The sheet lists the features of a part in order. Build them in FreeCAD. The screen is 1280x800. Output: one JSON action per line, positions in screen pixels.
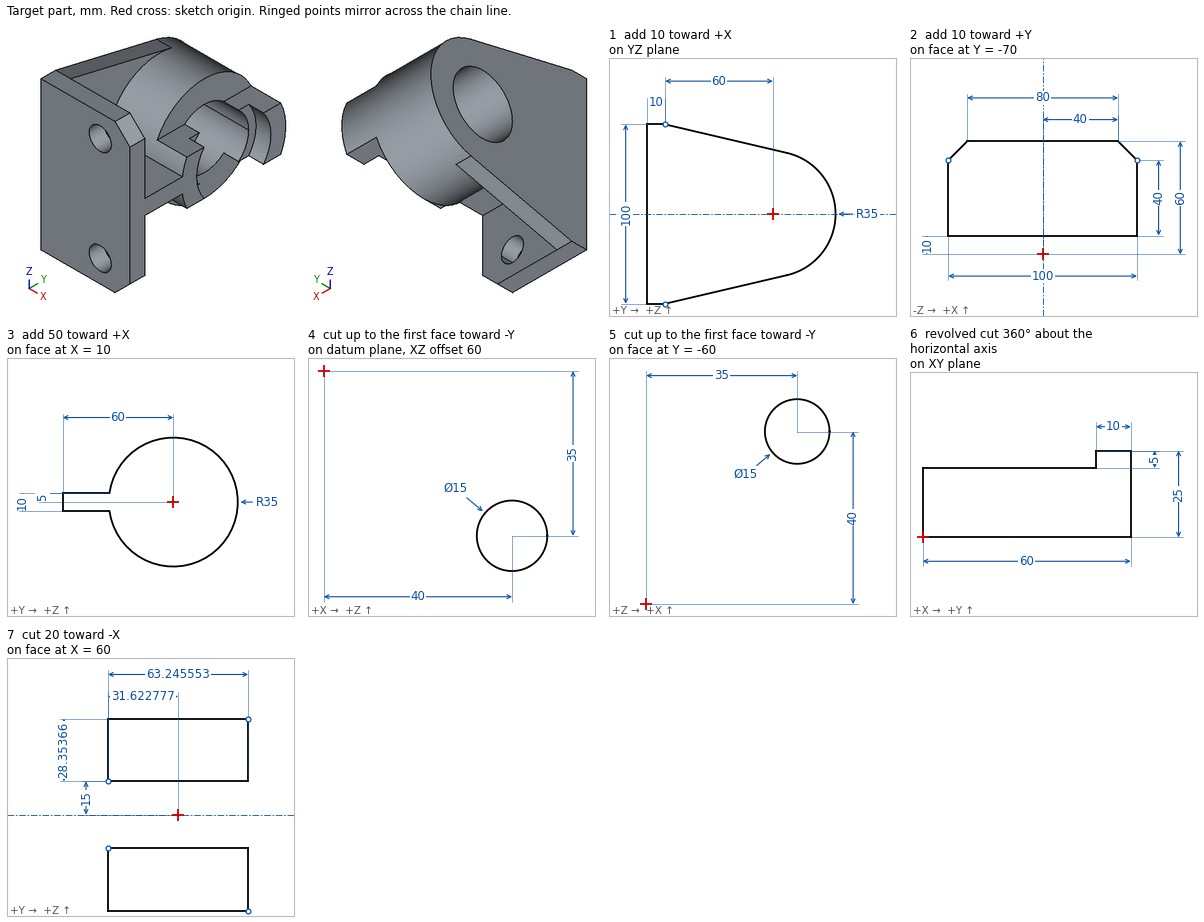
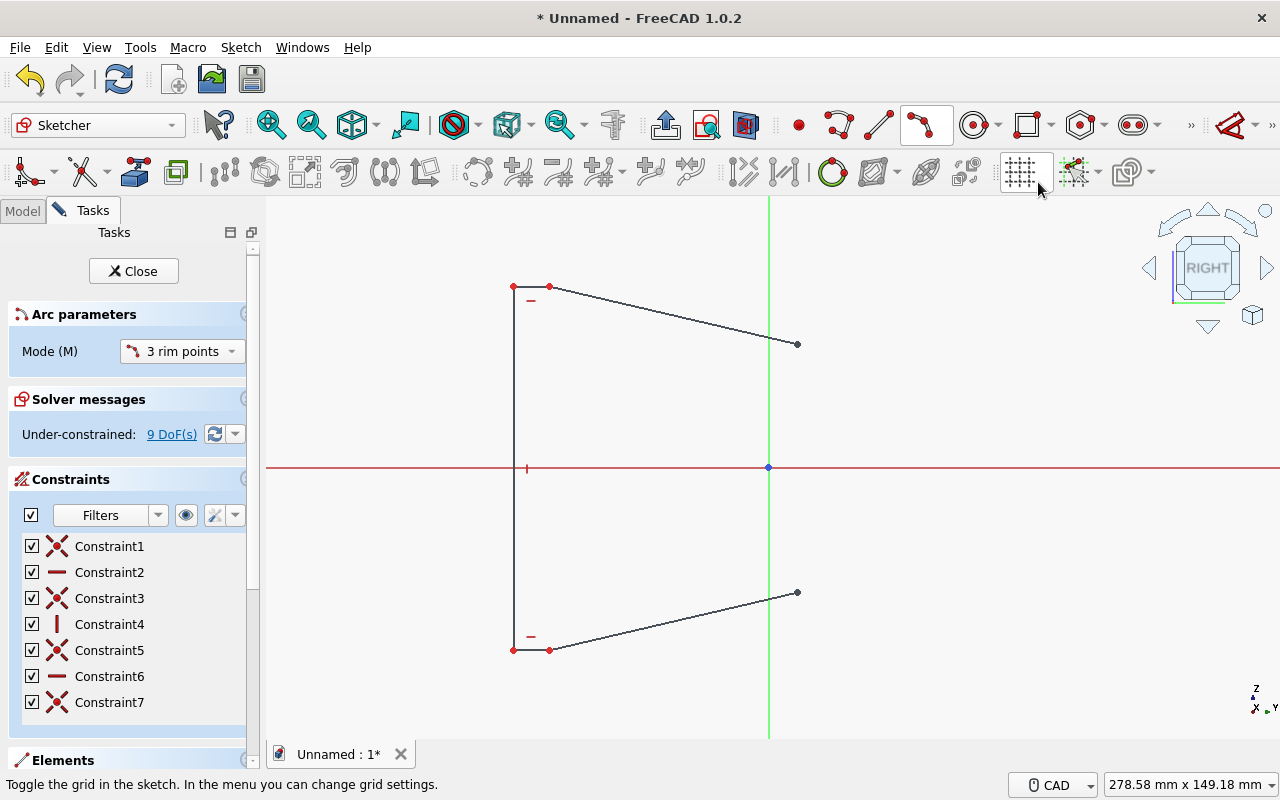
{"action": "left_click", "coordinate": [798, 593]}
{"action": "left_click", "coordinate": [798, 344]}
{"action": "left_click", "coordinate": [891, 501]}
{"action": "key", "text": "Escape"}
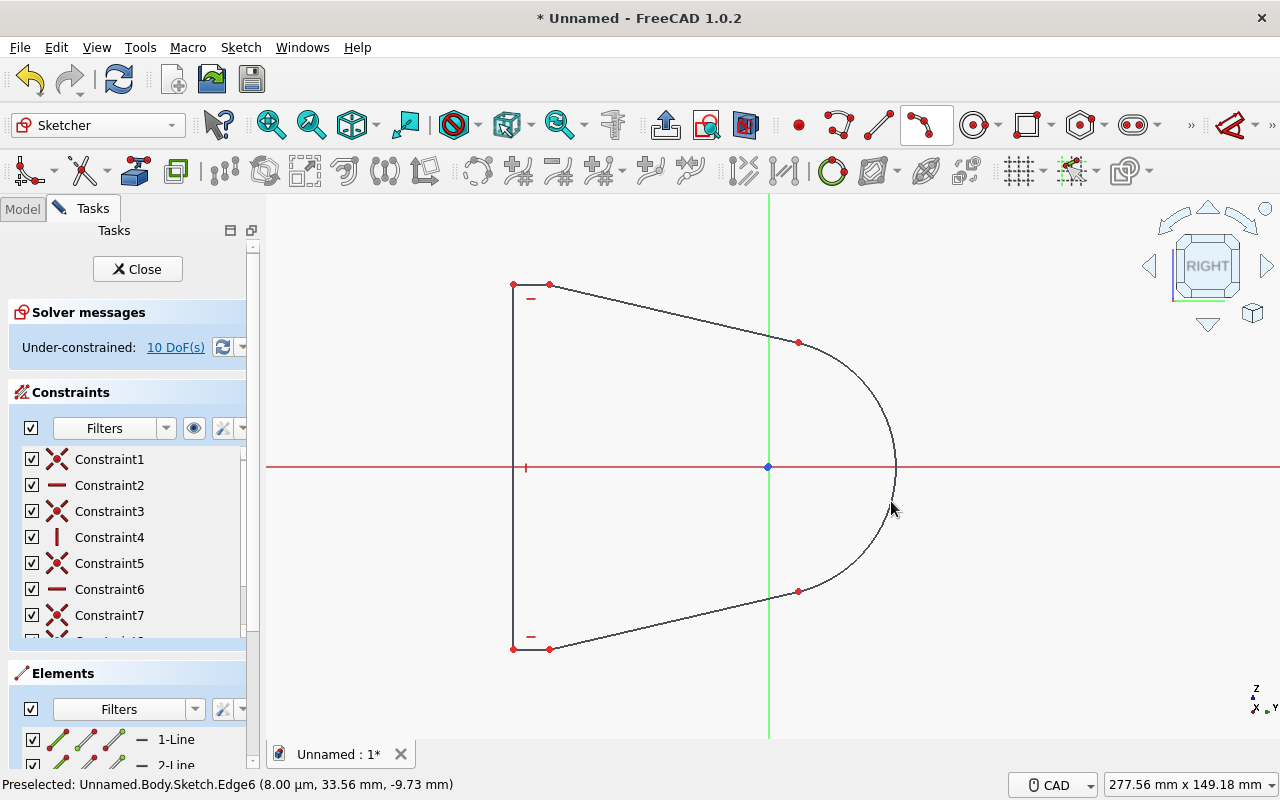
{"action": "left_click", "coordinate": [723, 326]}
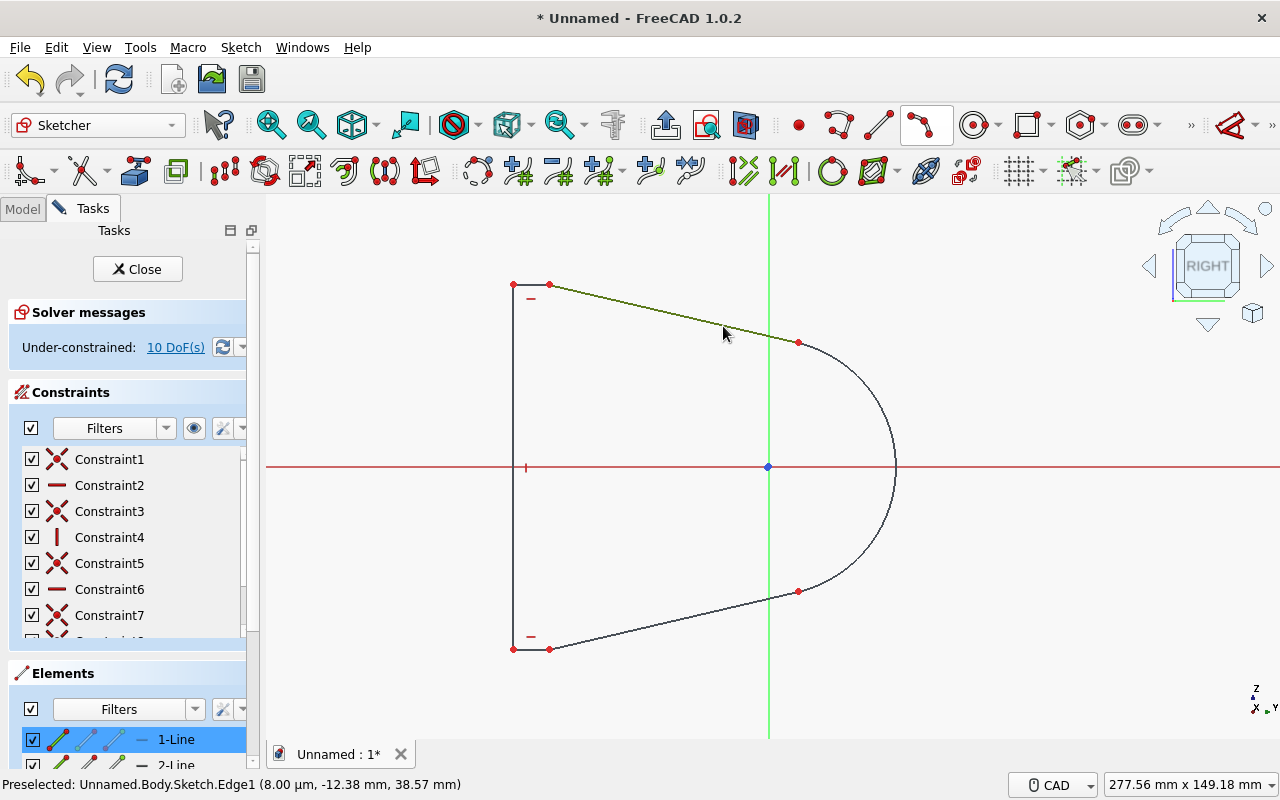
{"action": "left_click", "coordinate": [878, 533]}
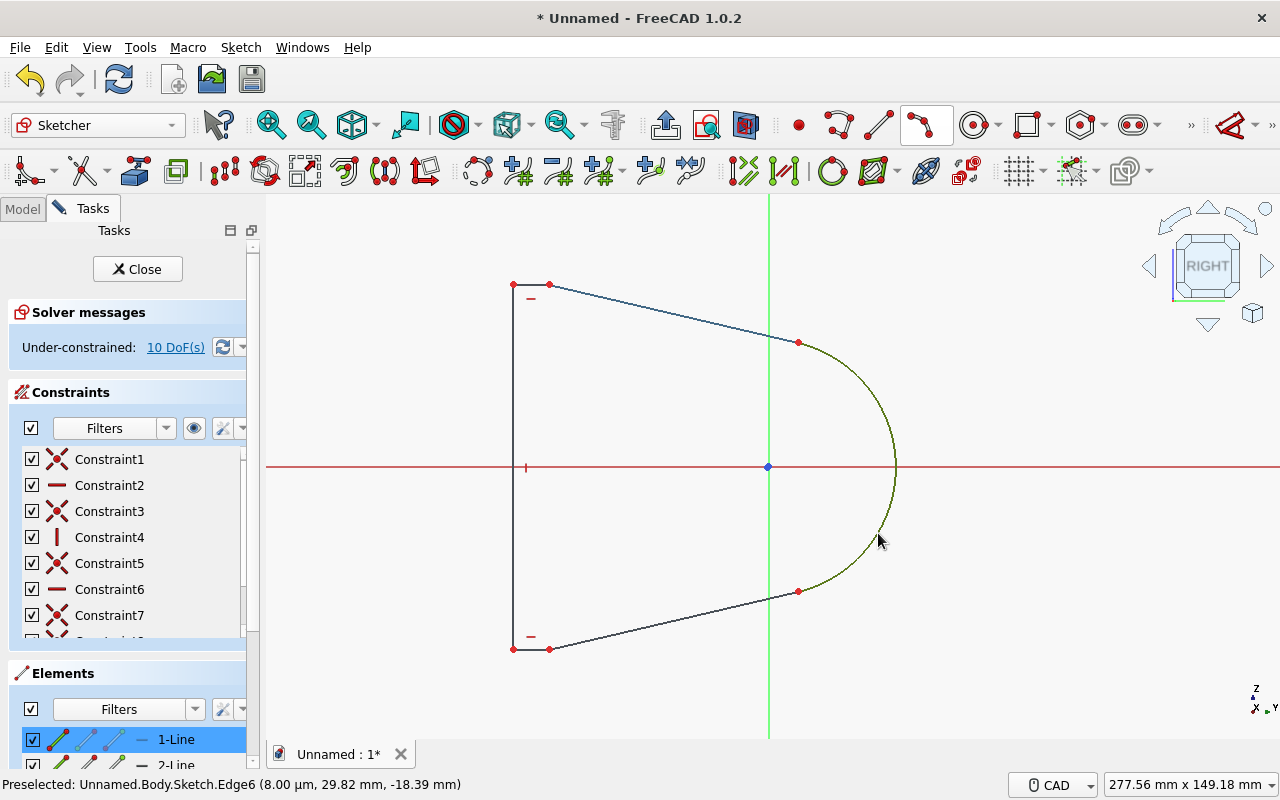
{"action": "key", "text": "t"}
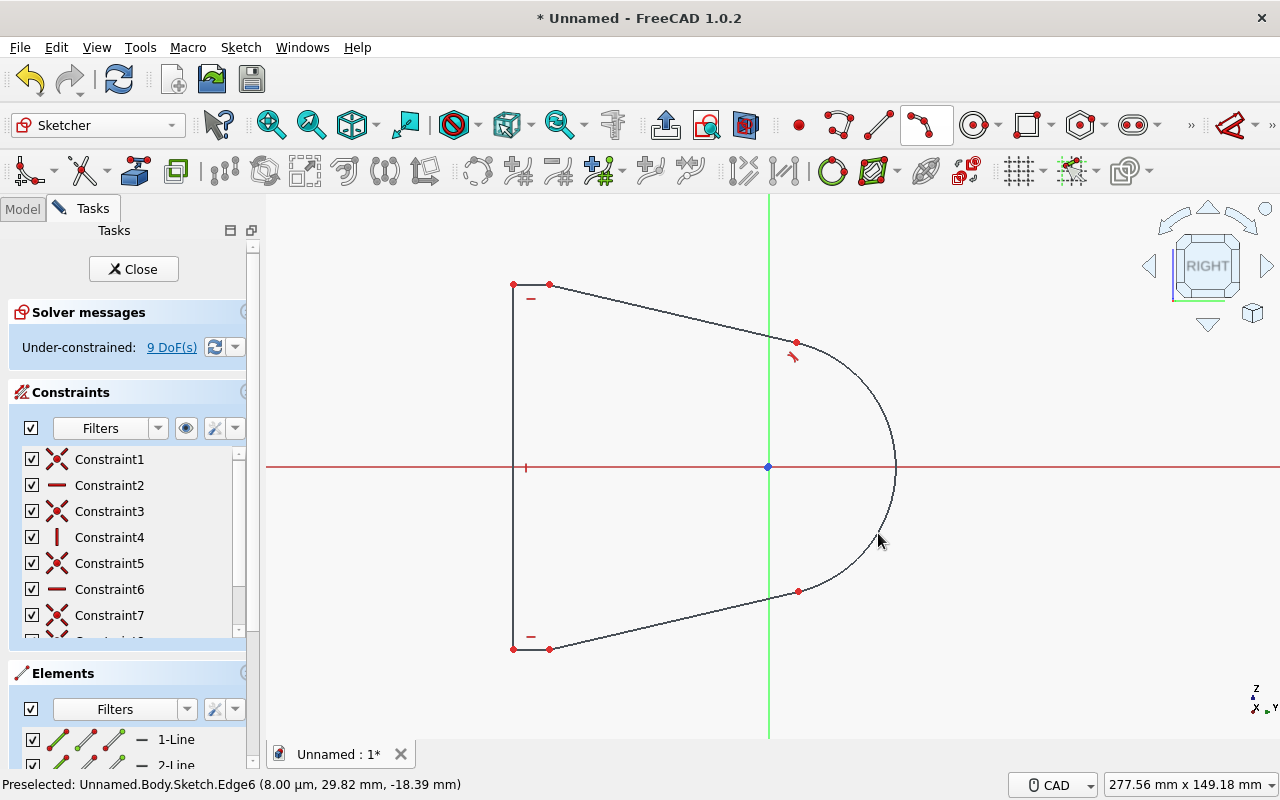
{"action": "left_click", "coordinate": [624, 633]}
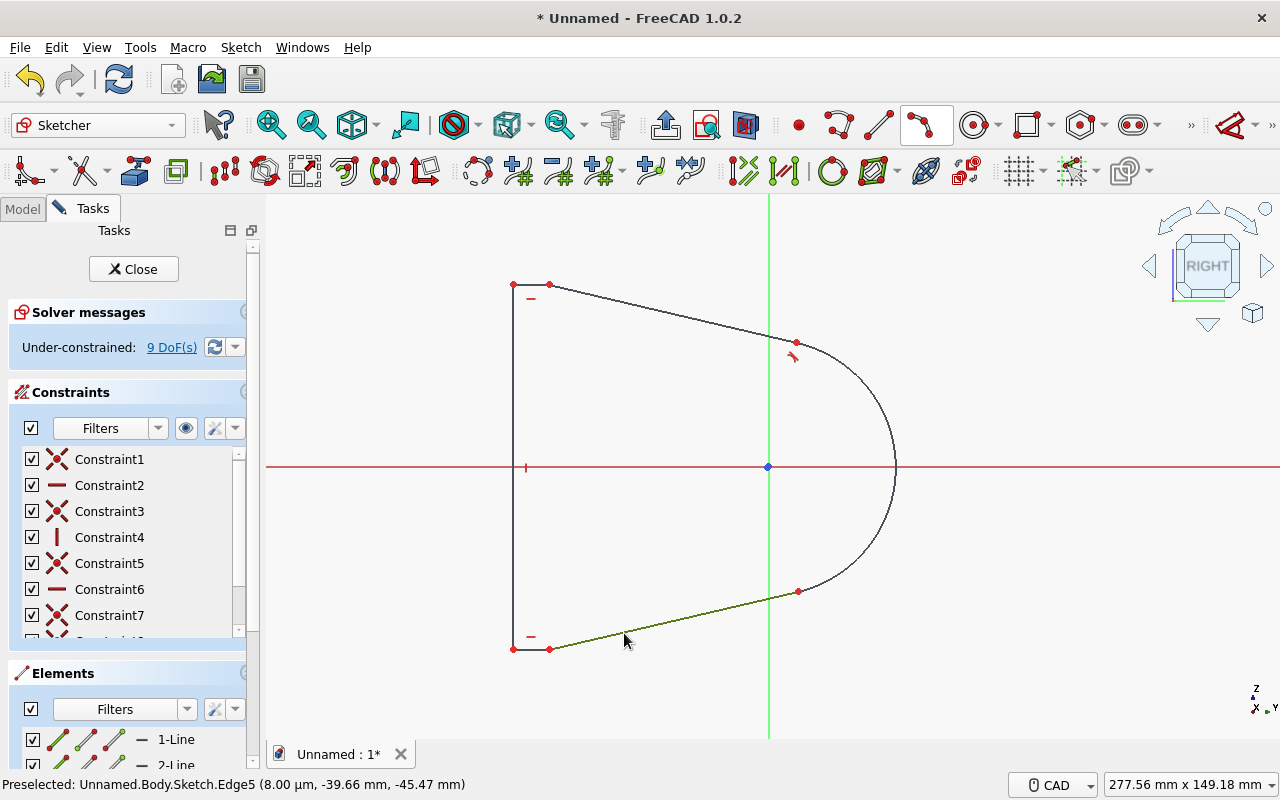
{"action": "left_click", "coordinate": [878, 532]}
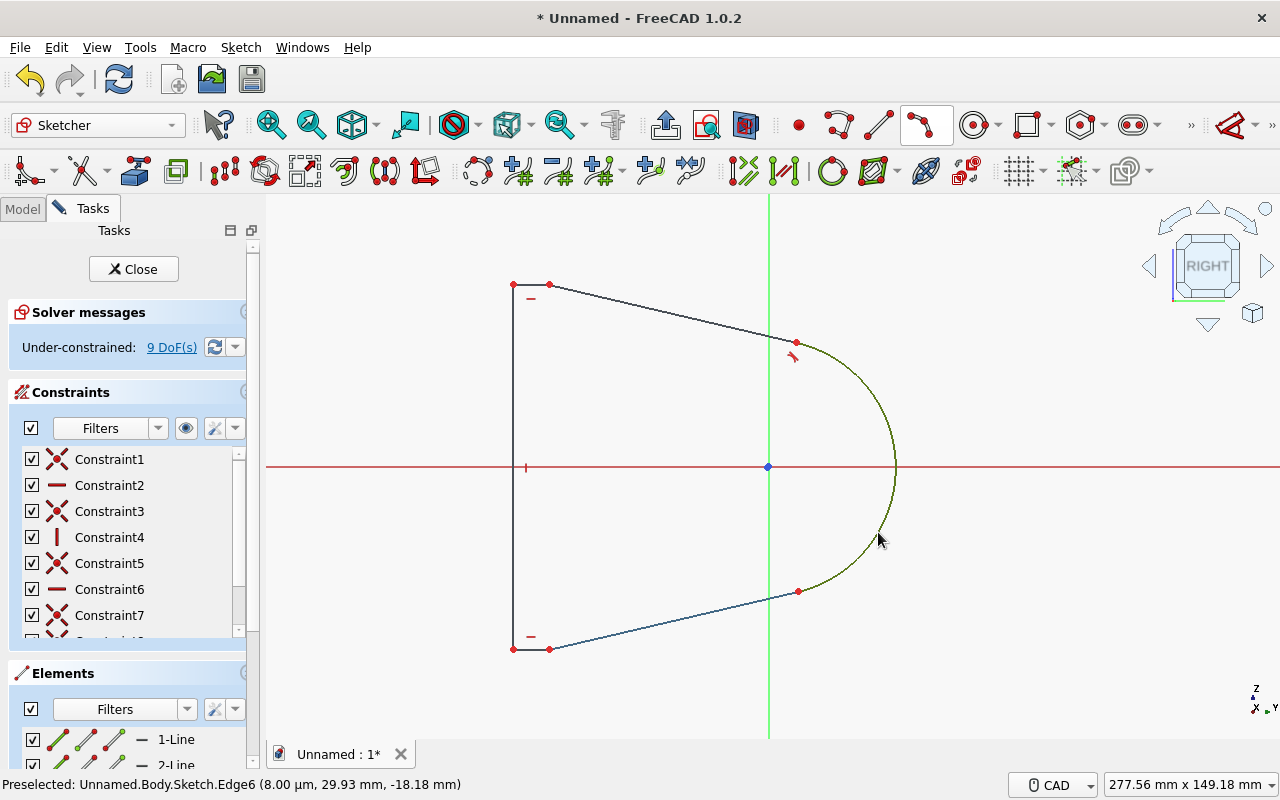
{"action": "key", "text": "t"}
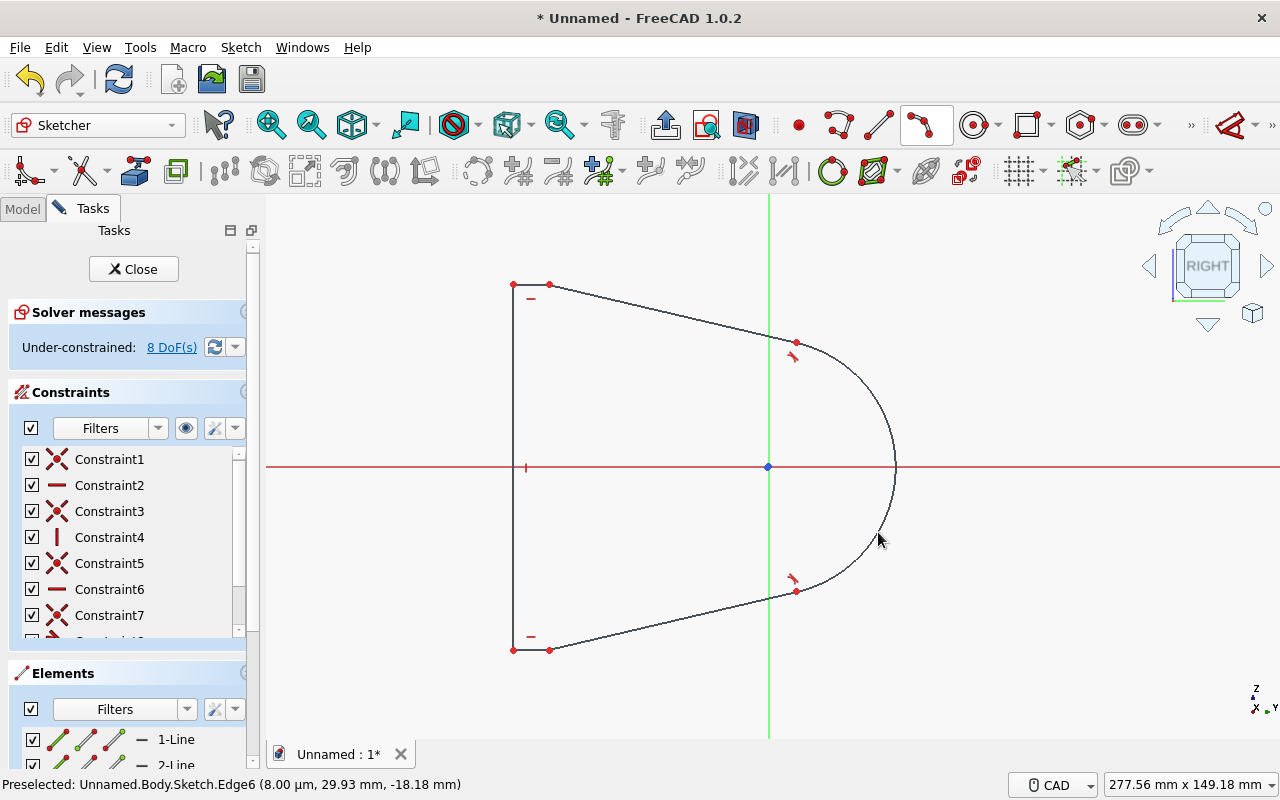
{"action": "left_click_drag", "start_coordinate": [758, 456], "coordinate": [779, 477]}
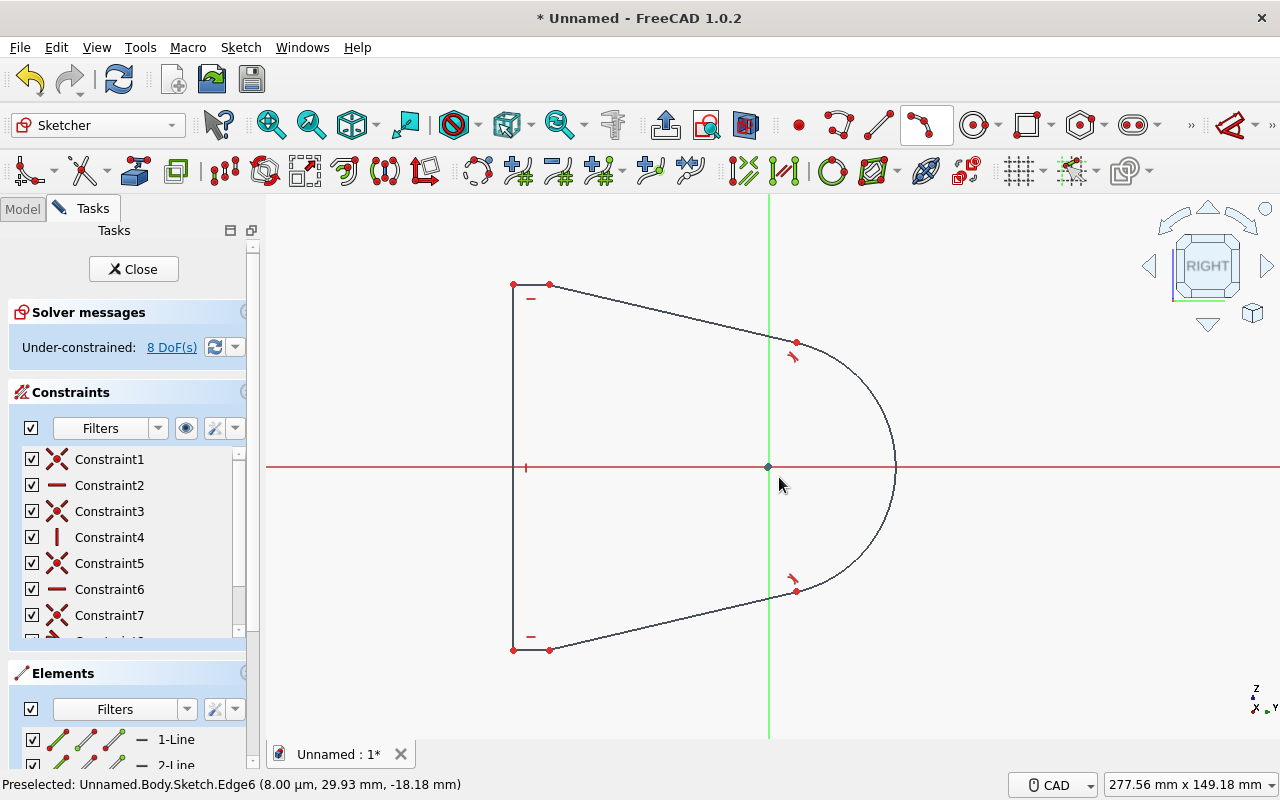
{"action": "key", "text": "c"}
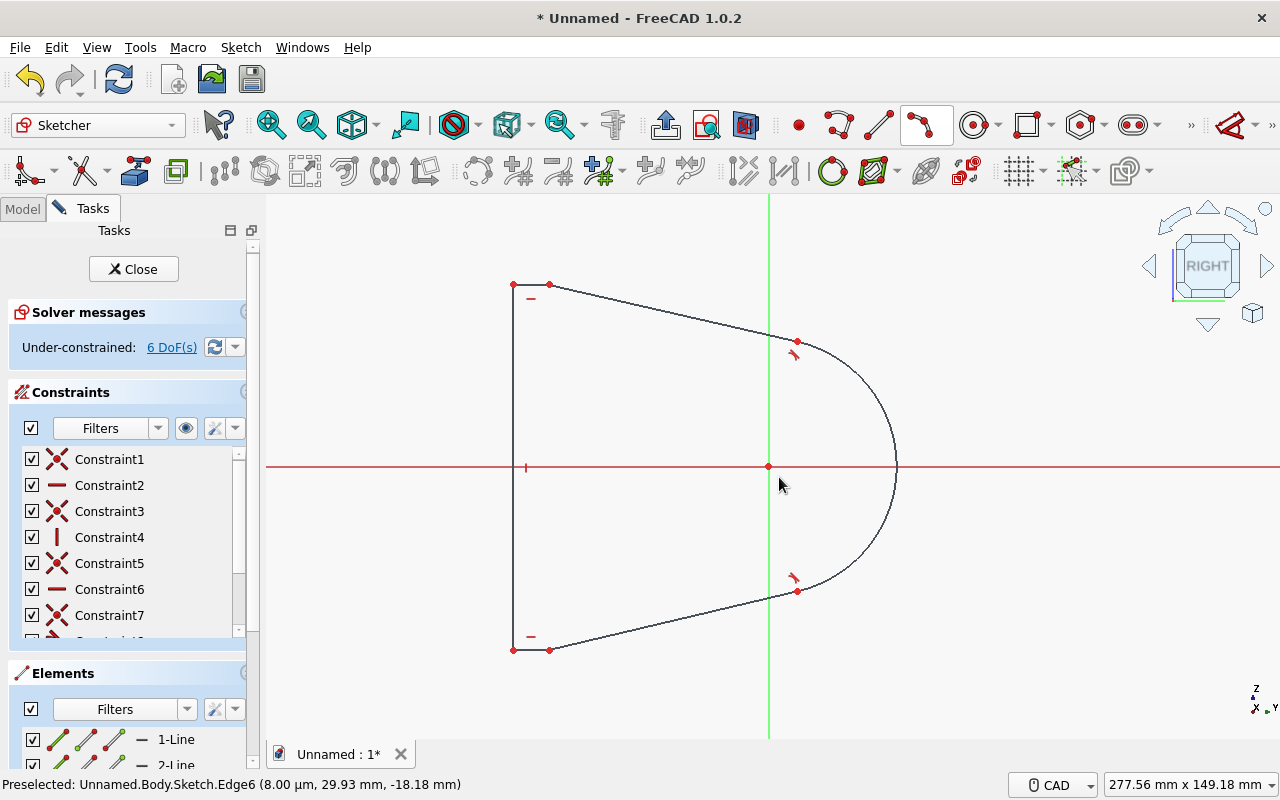
{"action": "left_click", "coordinate": [549, 285]}